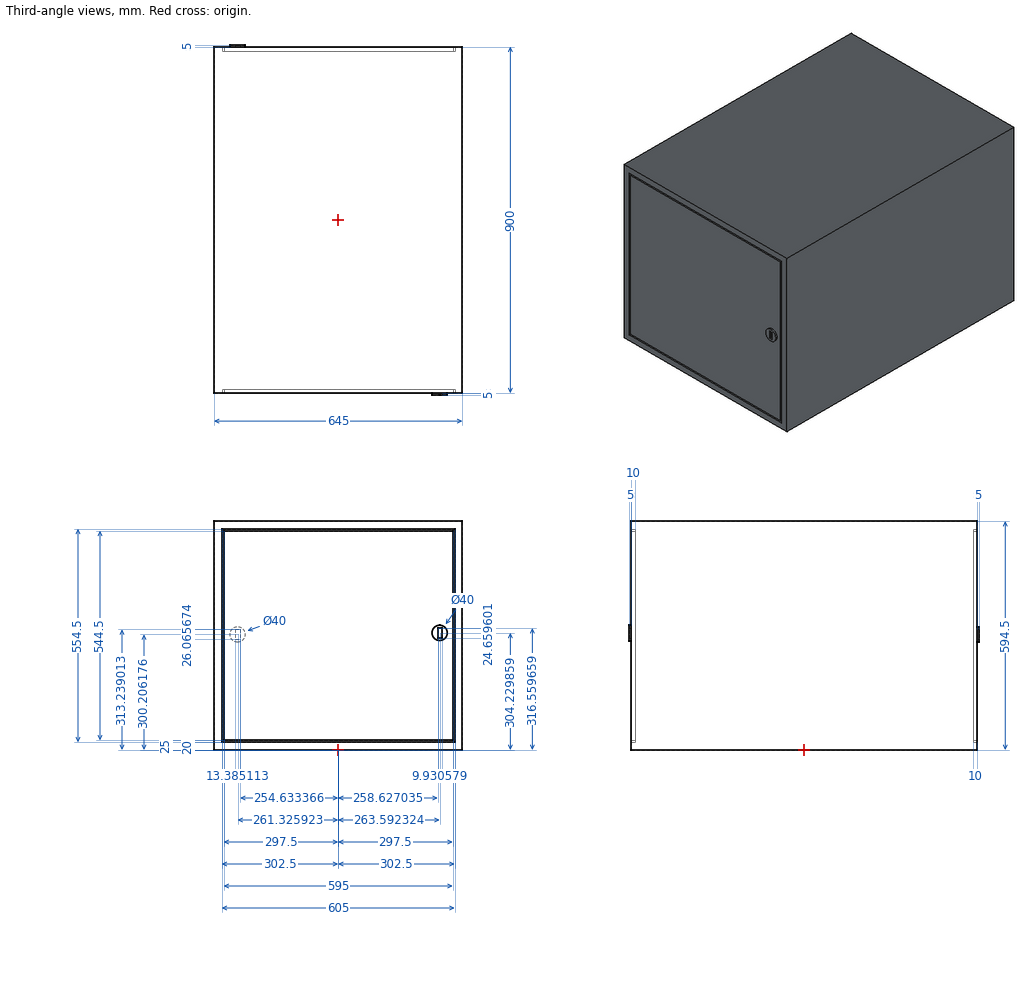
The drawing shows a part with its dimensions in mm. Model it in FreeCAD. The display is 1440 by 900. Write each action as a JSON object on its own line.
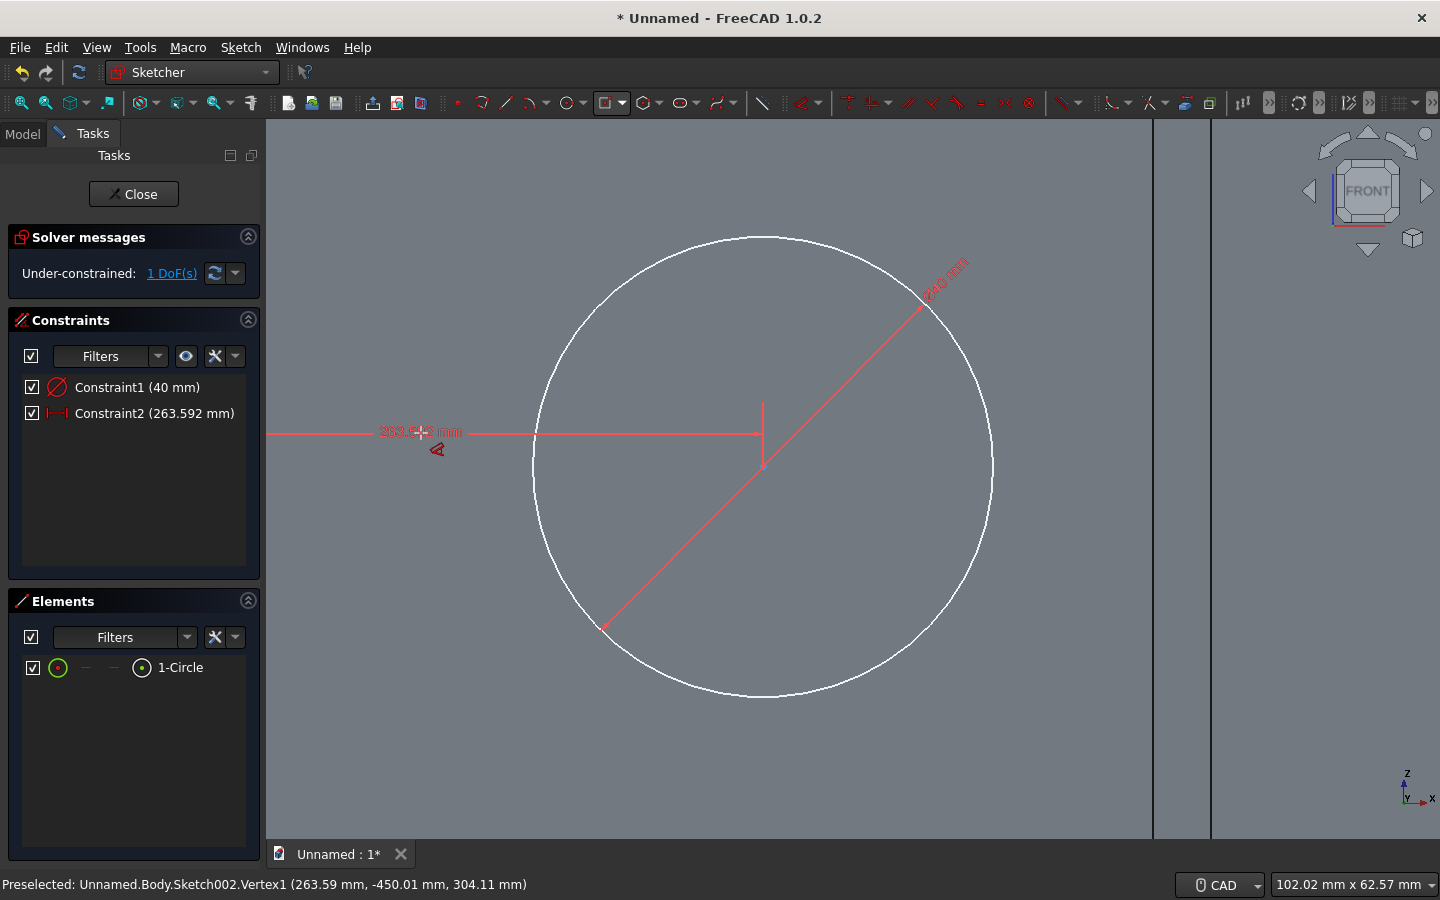
{"action": "left_click", "coordinate": [763, 467]}
{"action": "left_click", "coordinate": [797, 639]}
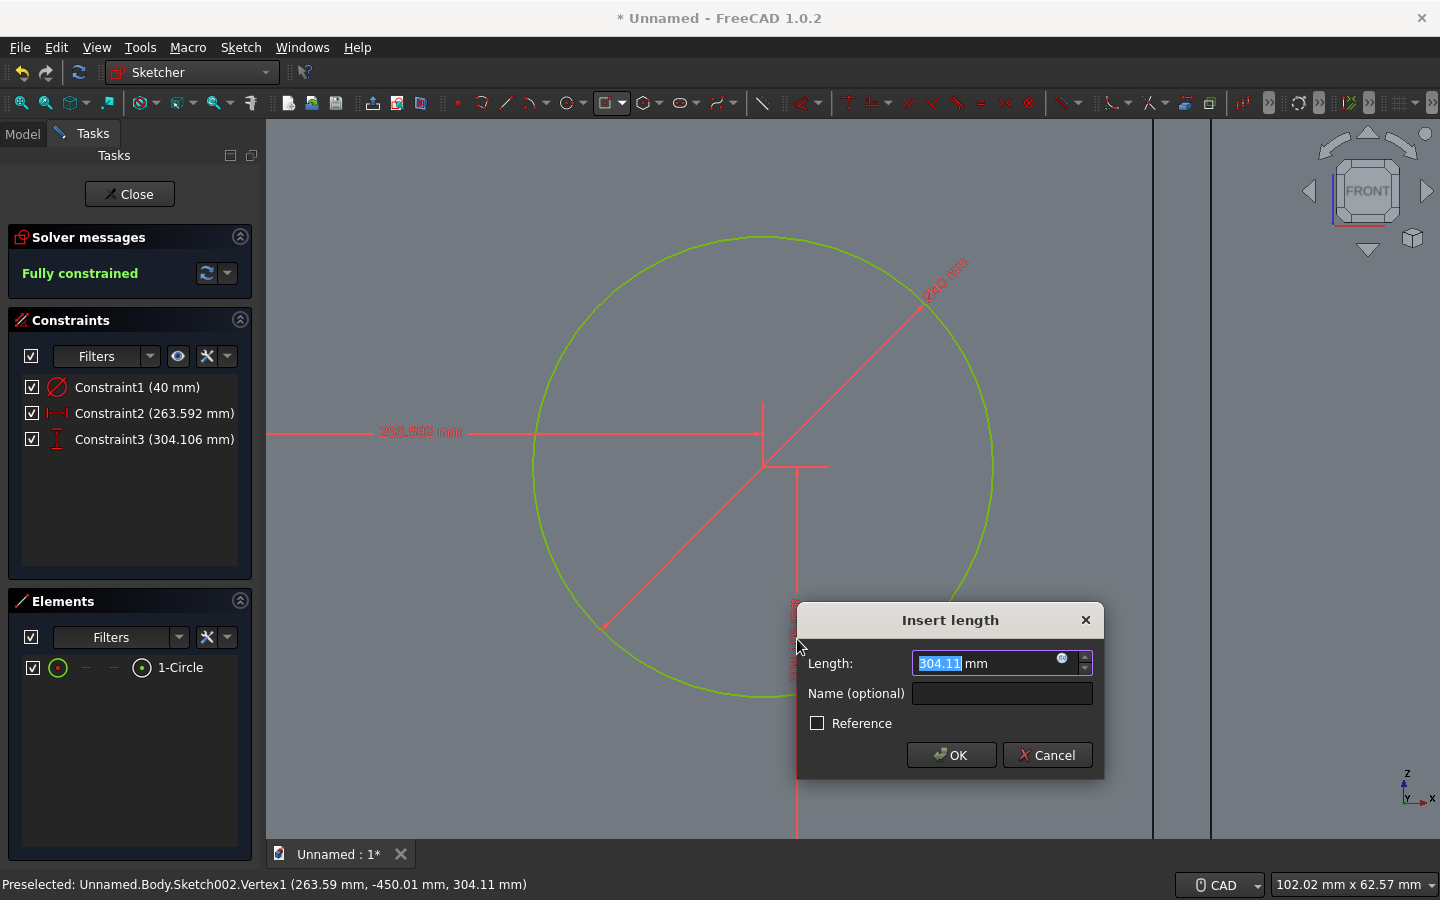
{"action": "type", "text": "304.229859"}
{"action": "key", "text": "Return"}
{"action": "key", "text": "Escape"}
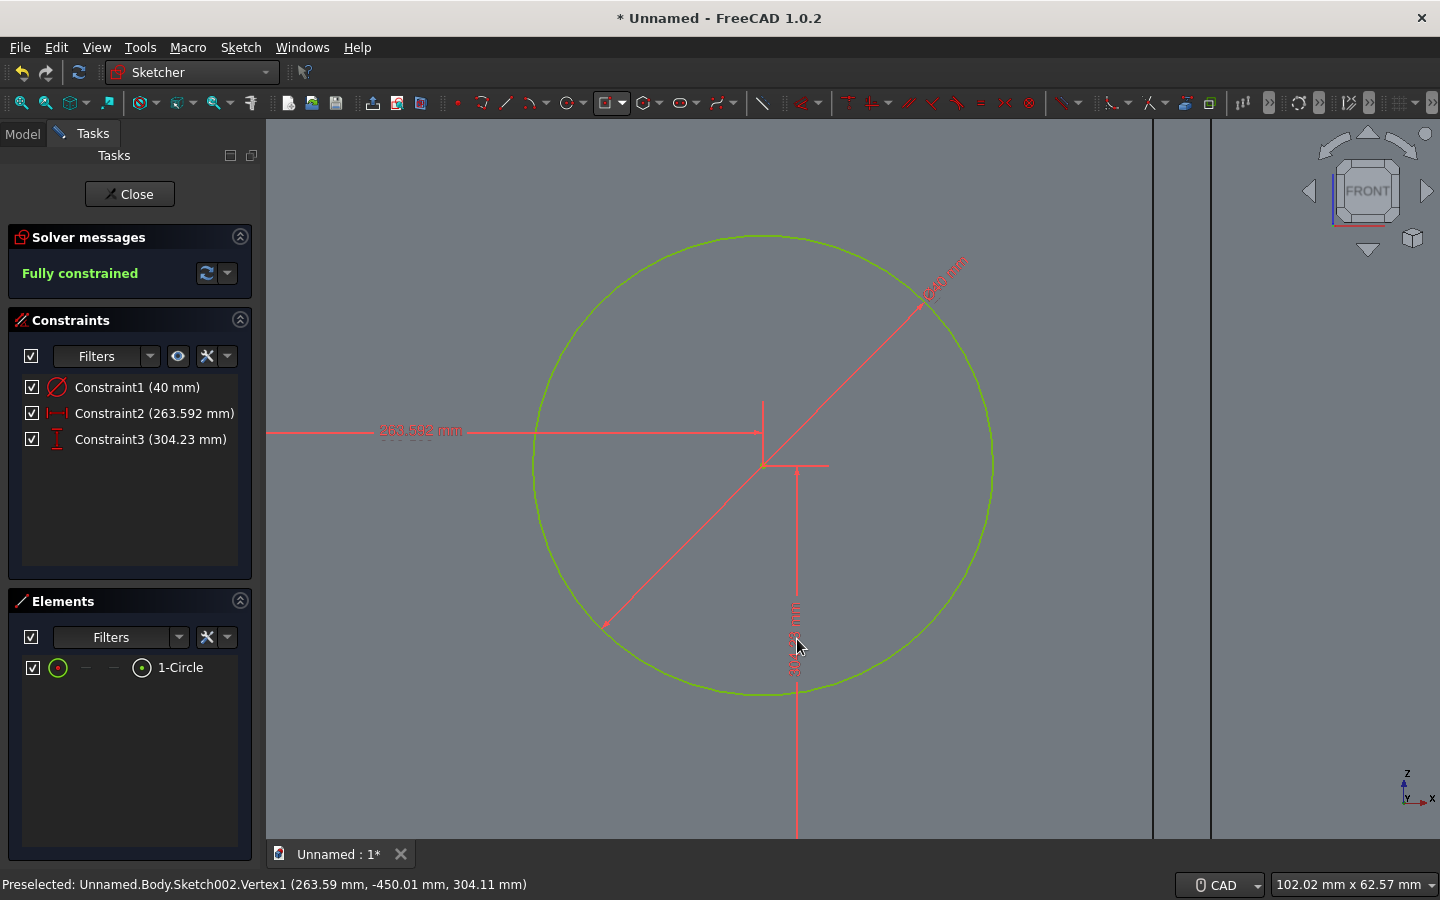
{"action": "left_click", "coordinate": [130, 194]}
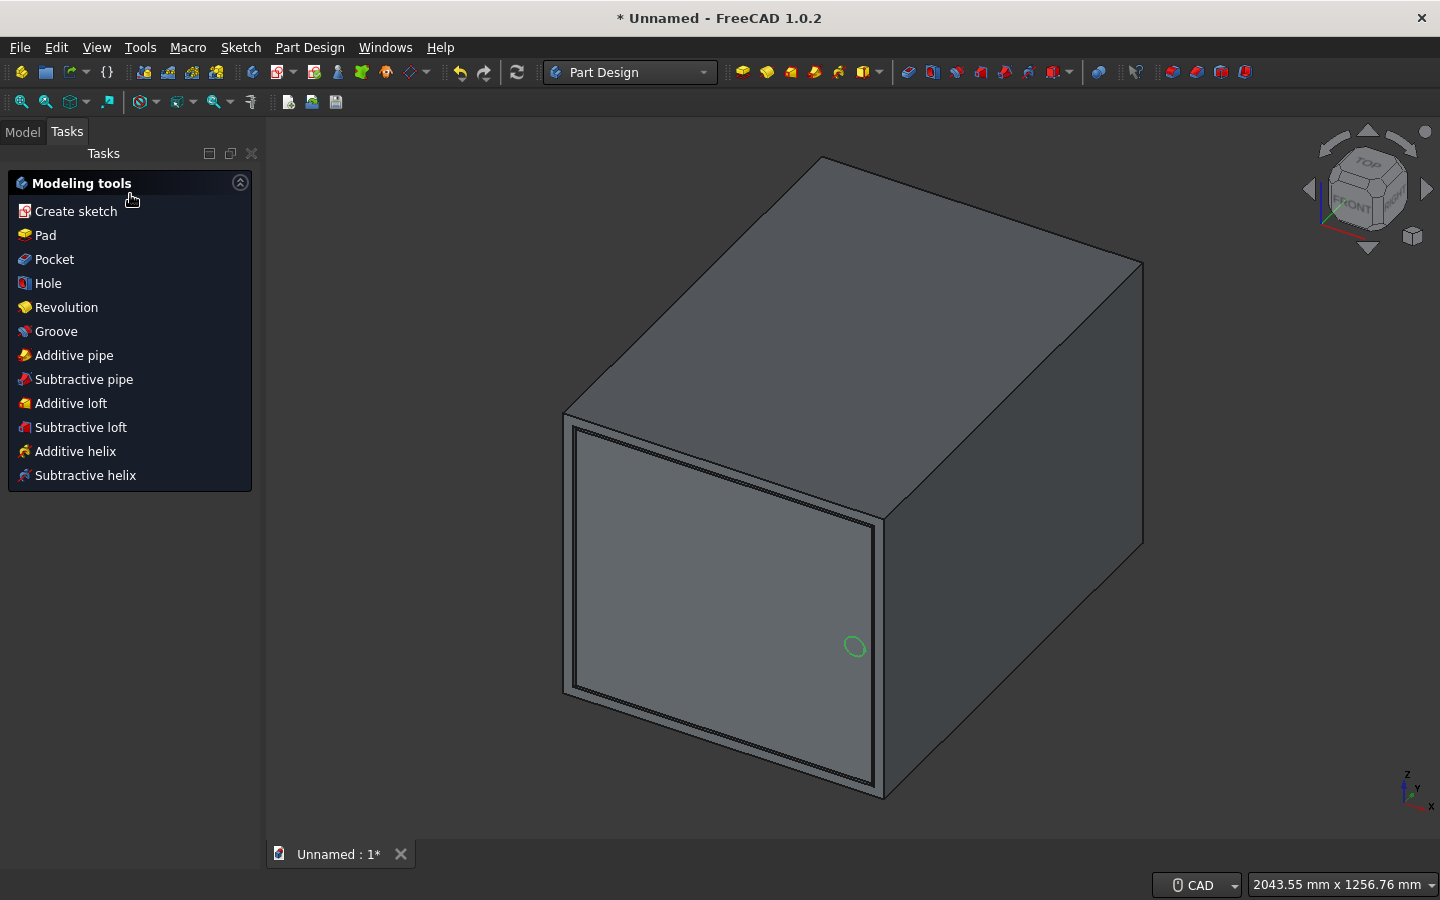
{"action": "left_click", "coordinate": [744, 72]}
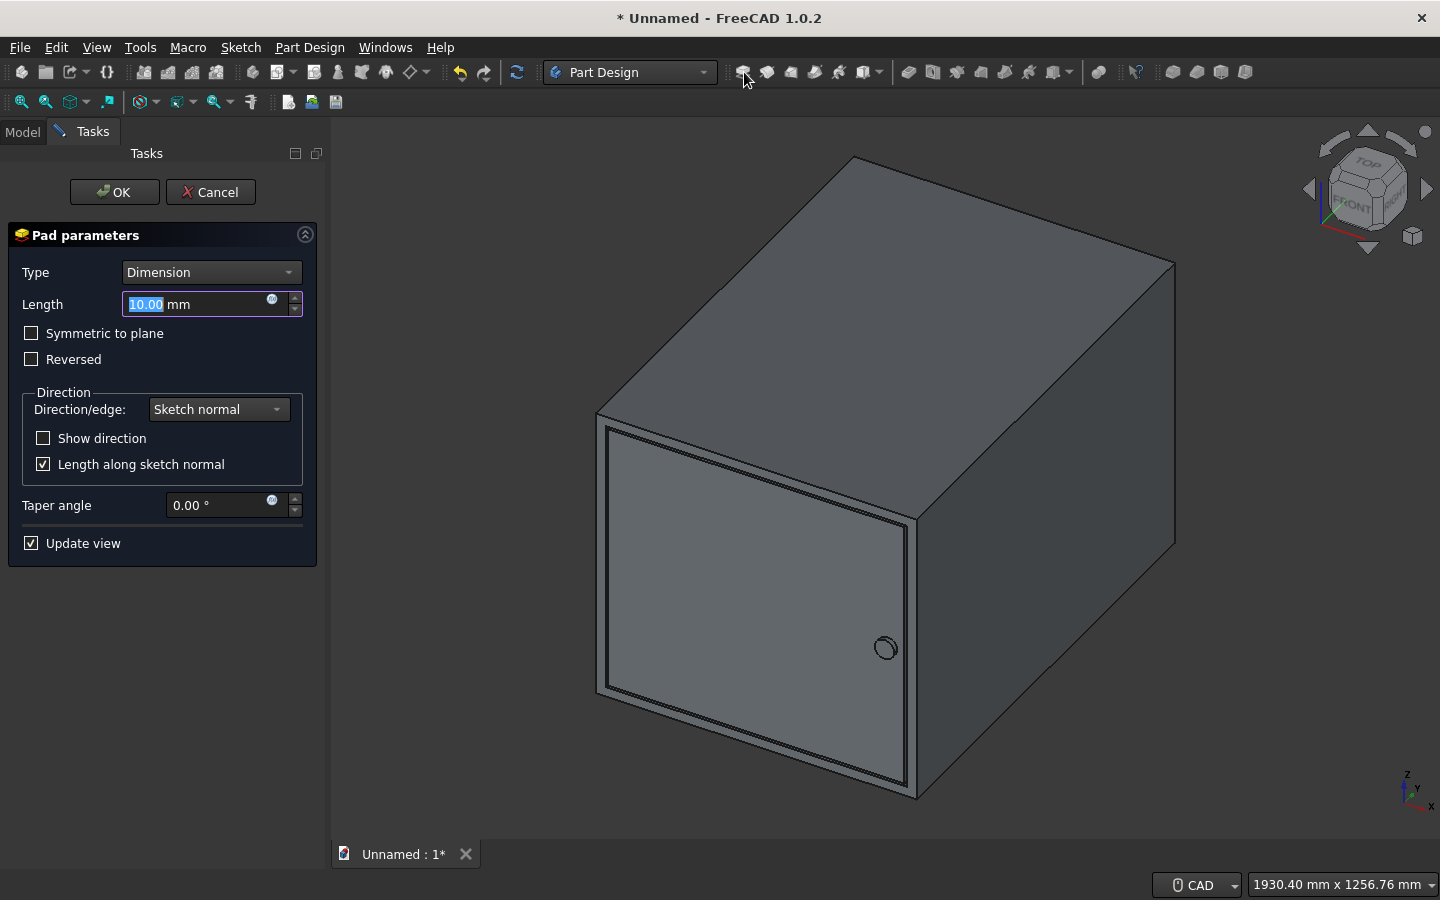
{"action": "type", "text": "5"}
{"action": "key", "text": "Tab"}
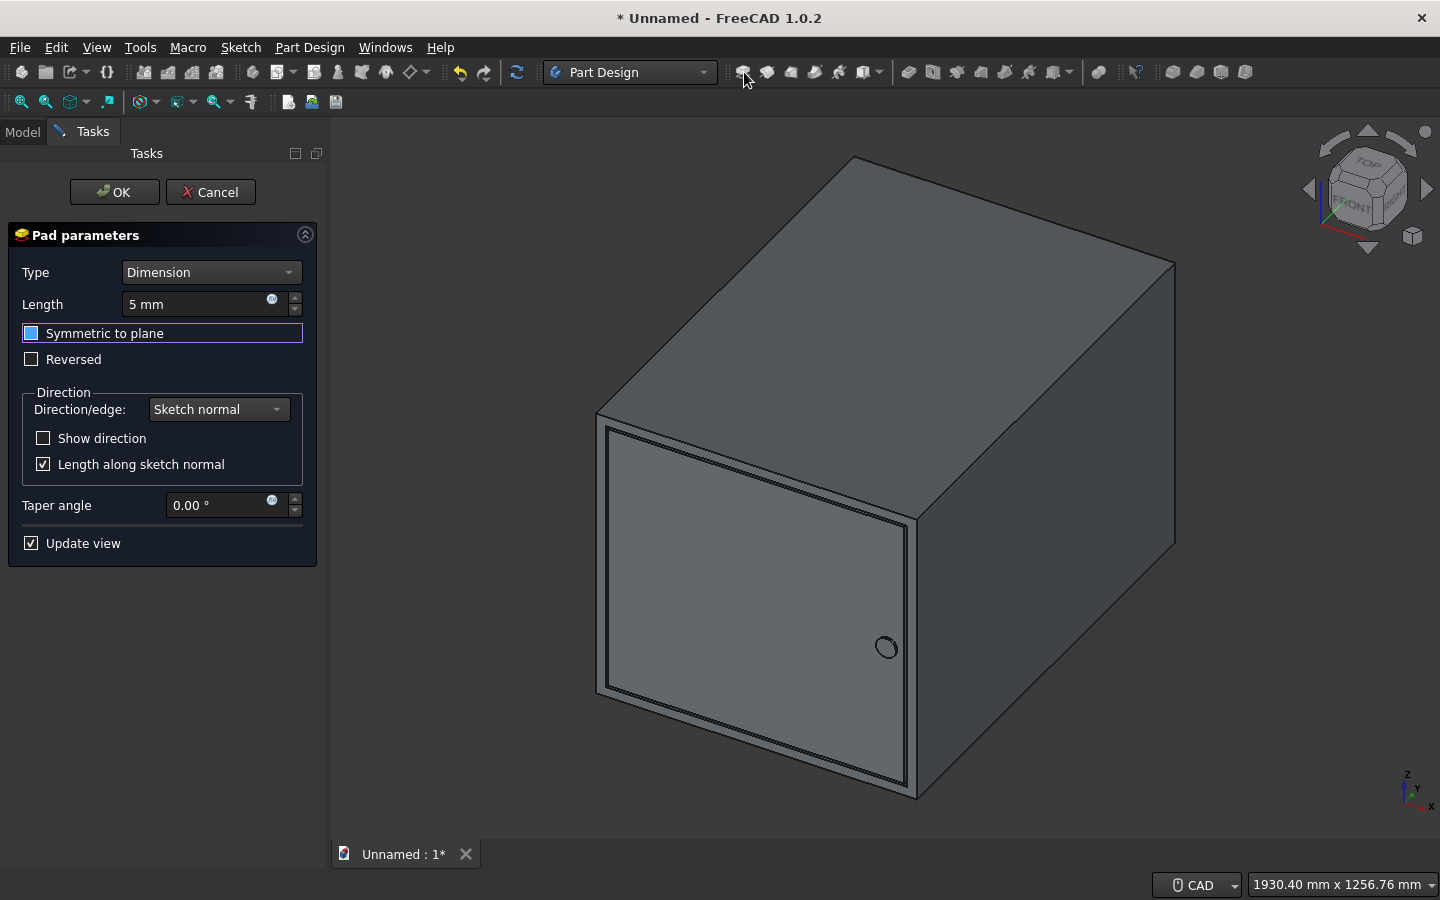
{"action": "left_click", "coordinate": [115, 192]}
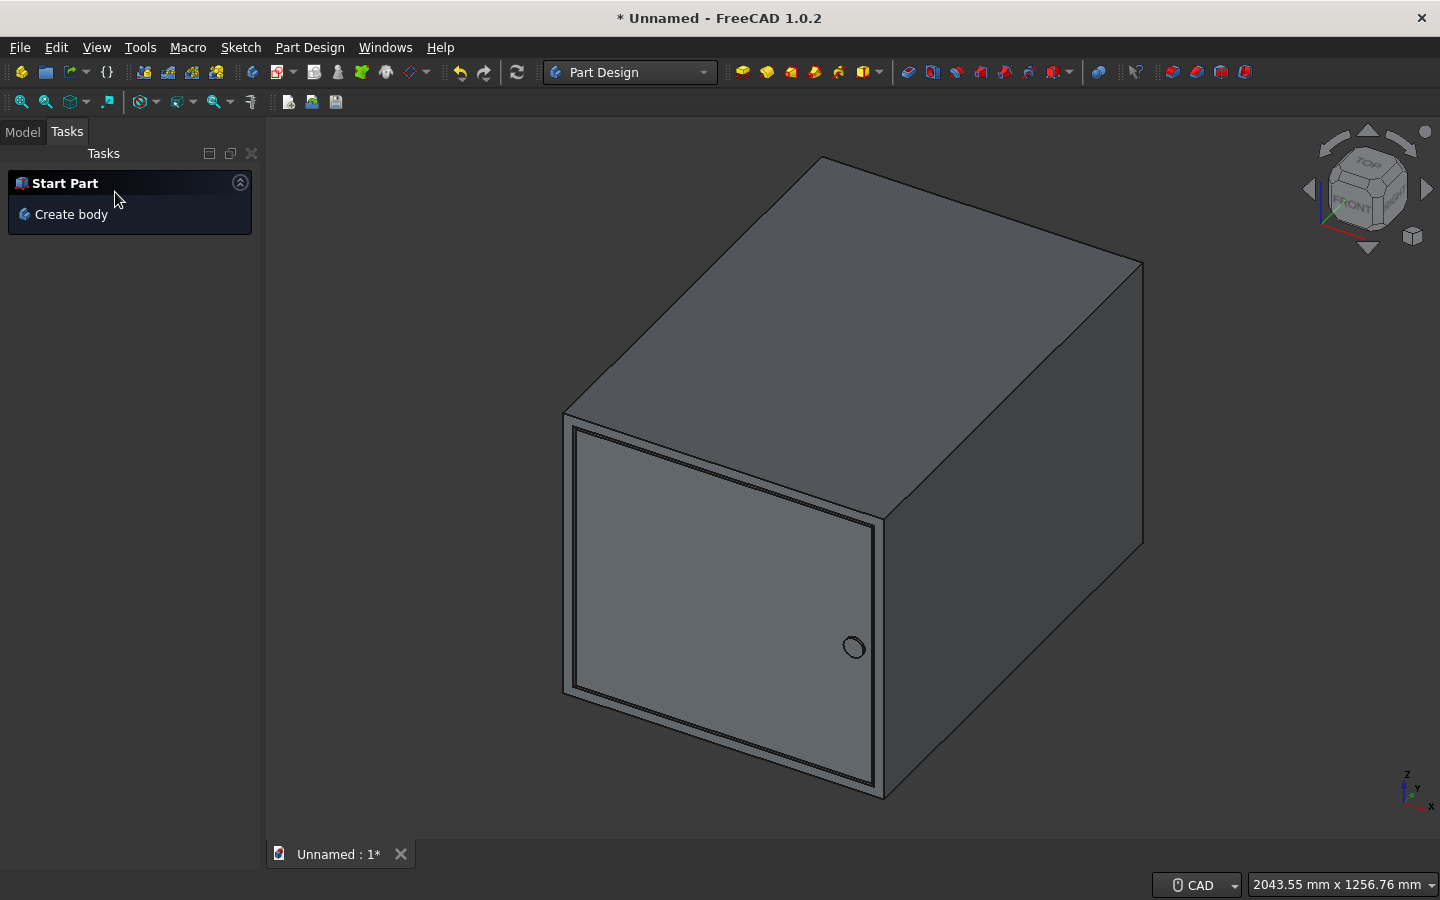
{"action": "left_click", "coordinate": [853, 650]}